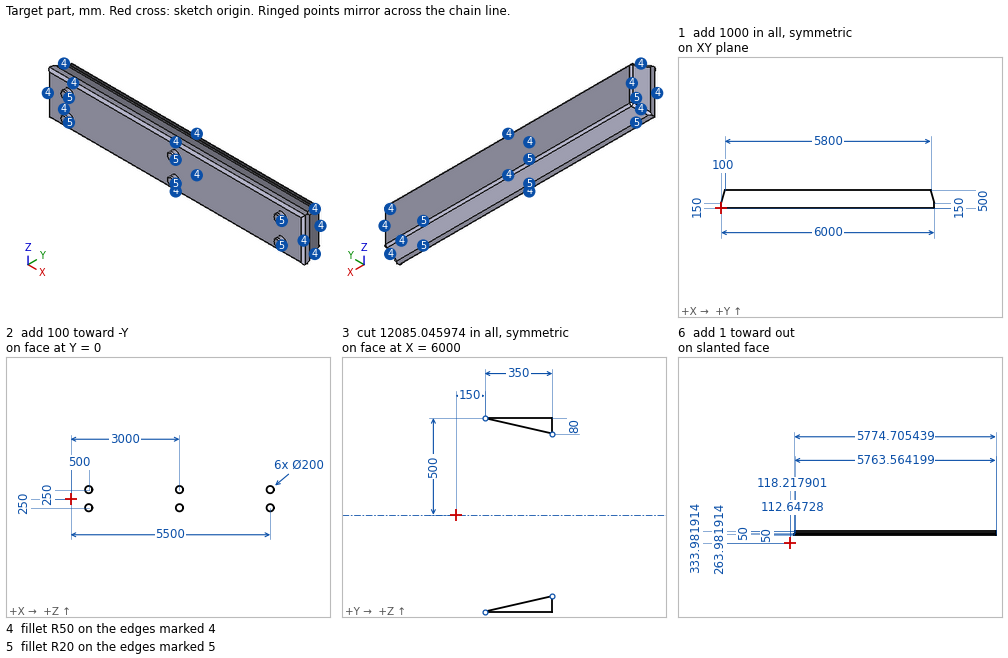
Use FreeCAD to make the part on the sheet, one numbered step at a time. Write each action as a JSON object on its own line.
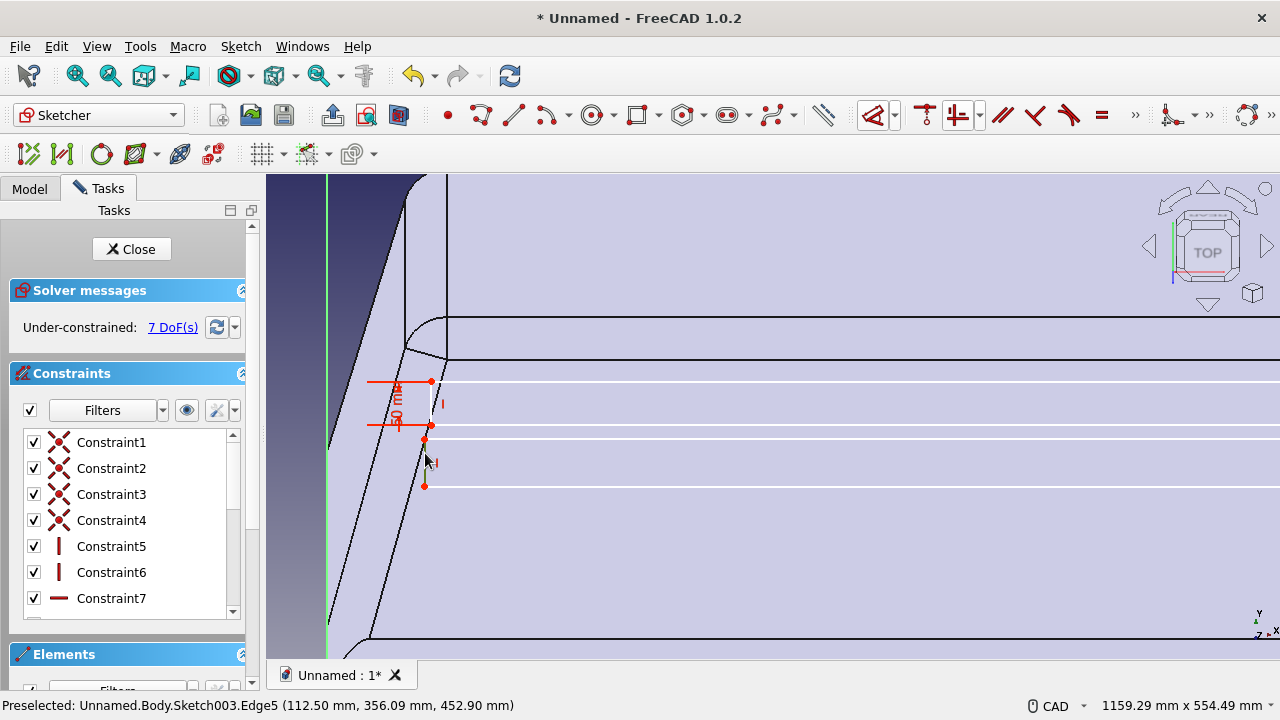
{"action": "left_click", "coordinate": [894, 116]}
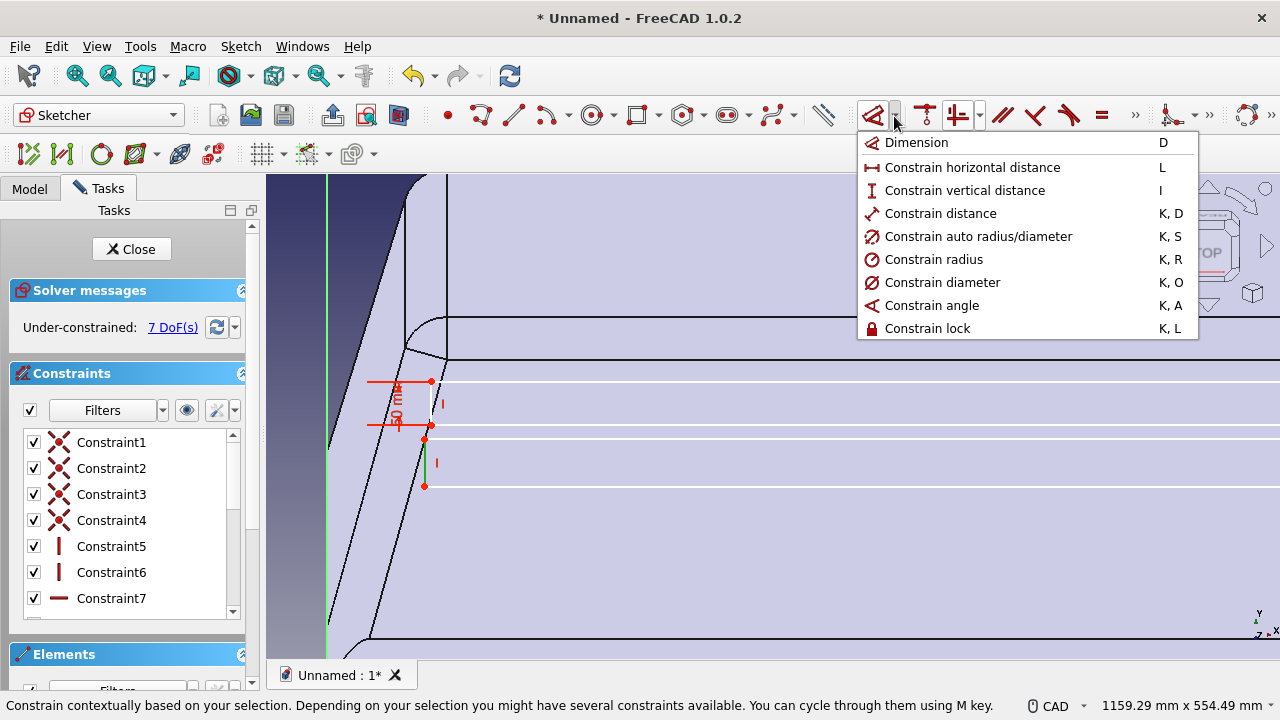
{"action": "left_click", "coordinate": [1028, 190]}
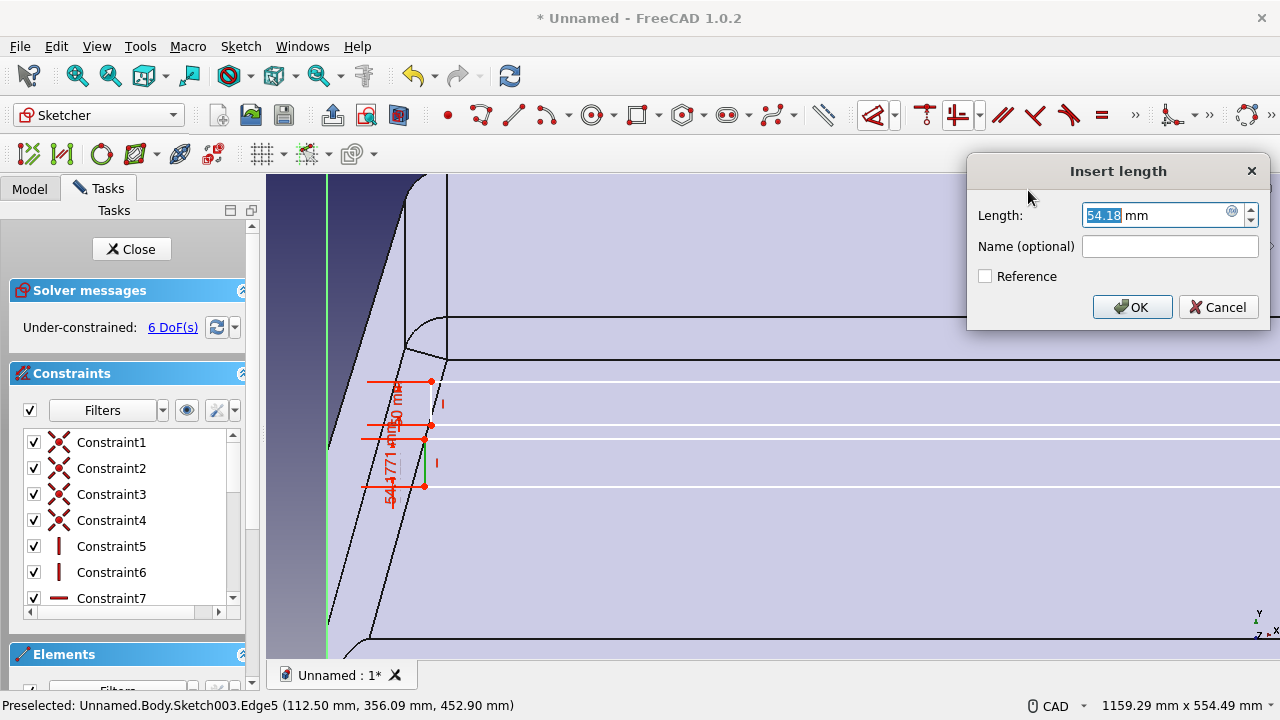
{"action": "type", "text": "50"}
{"action": "key", "text": "Return"}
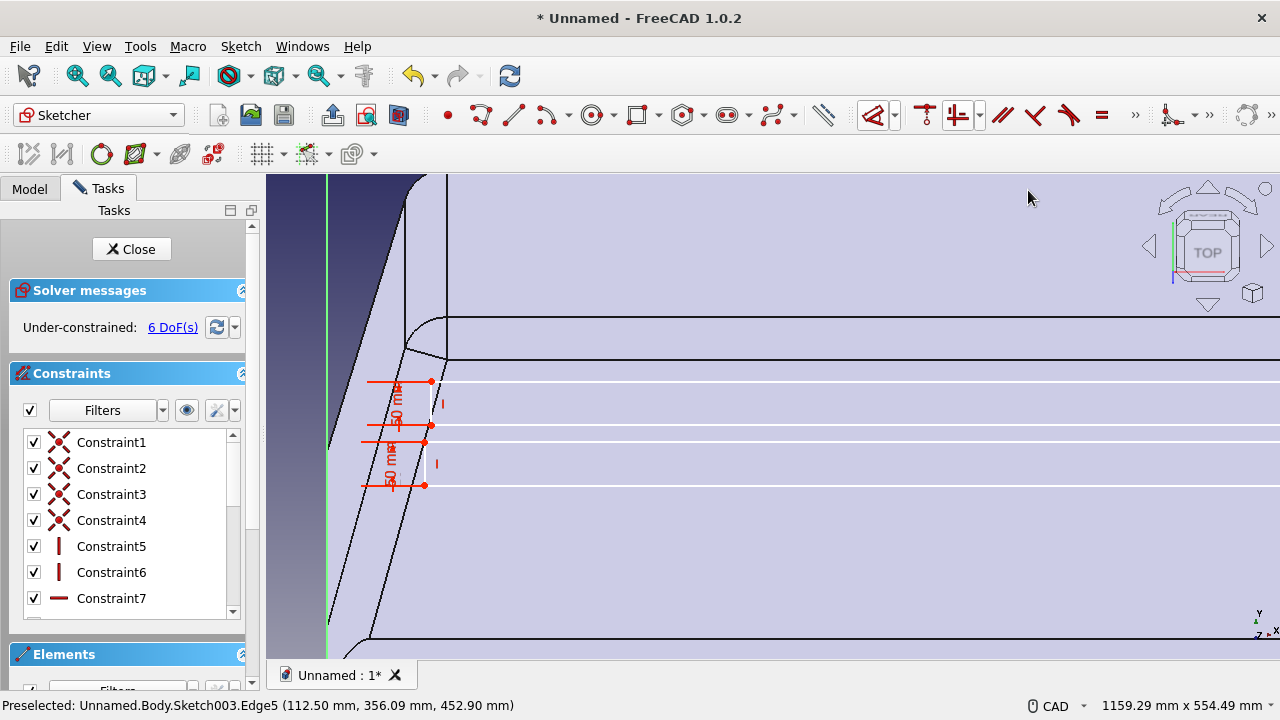
{"action": "left_click", "coordinate": [425, 442]}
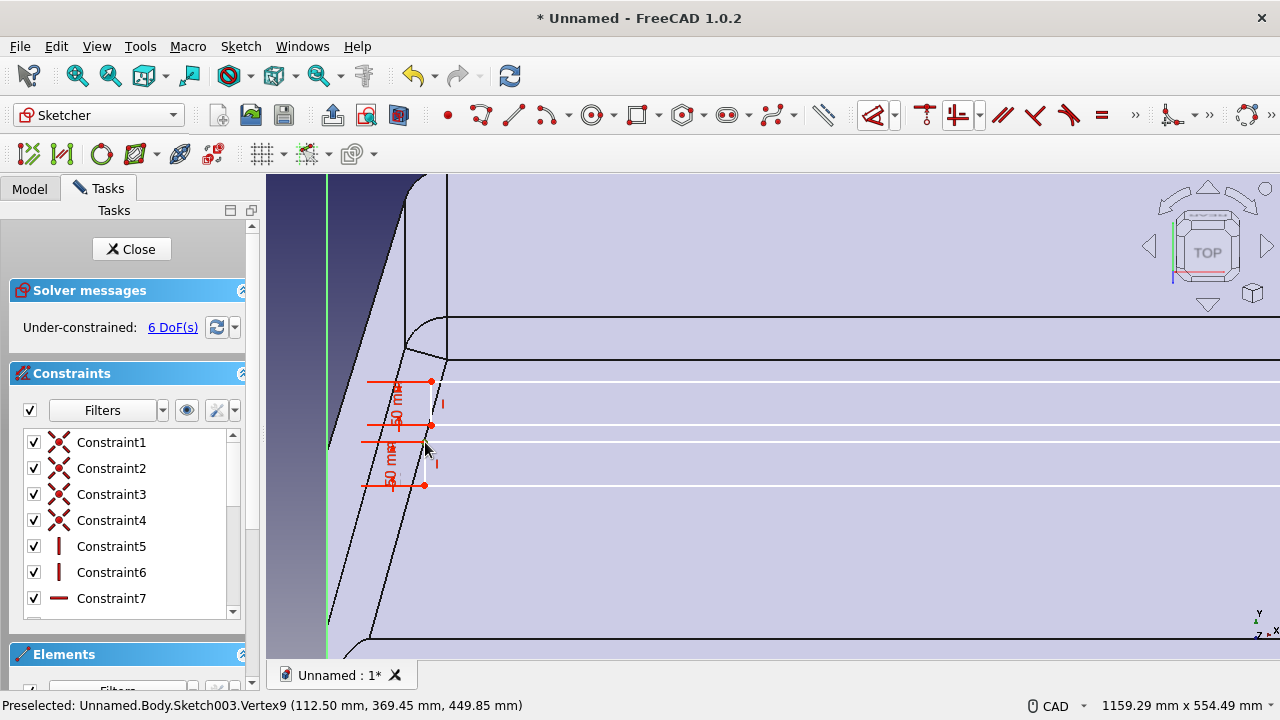
{"action": "key", "text": "l"}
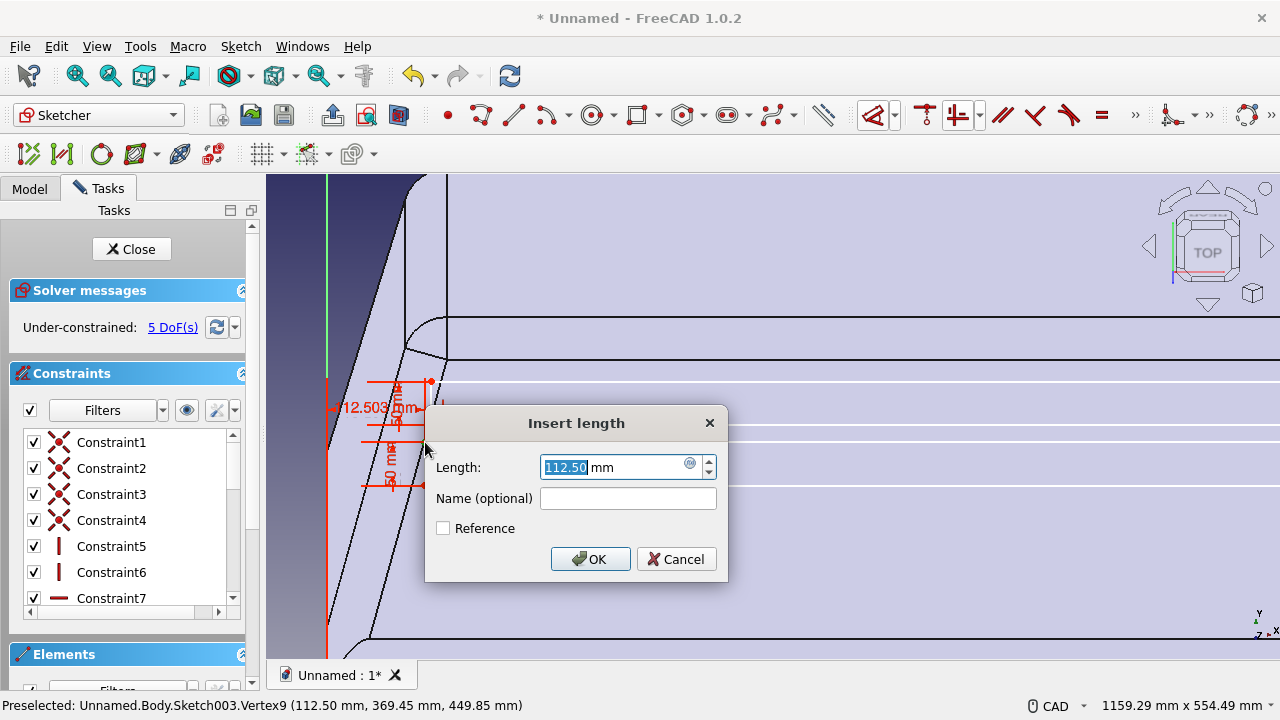
{"action": "type", "text": "112.64728"}
{"action": "key", "text": "Return"}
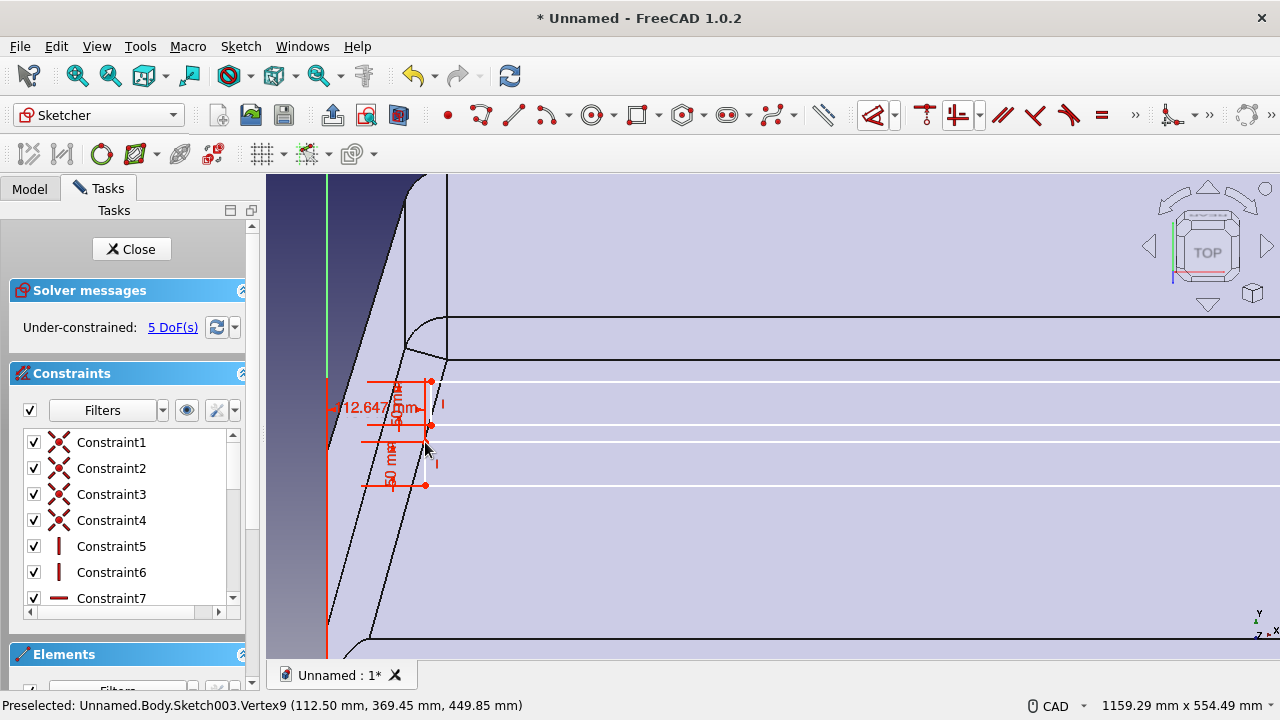
{"action": "scroll", "coordinate": [431, 403], "scroll_direction": "down", "scroll_amount": 11}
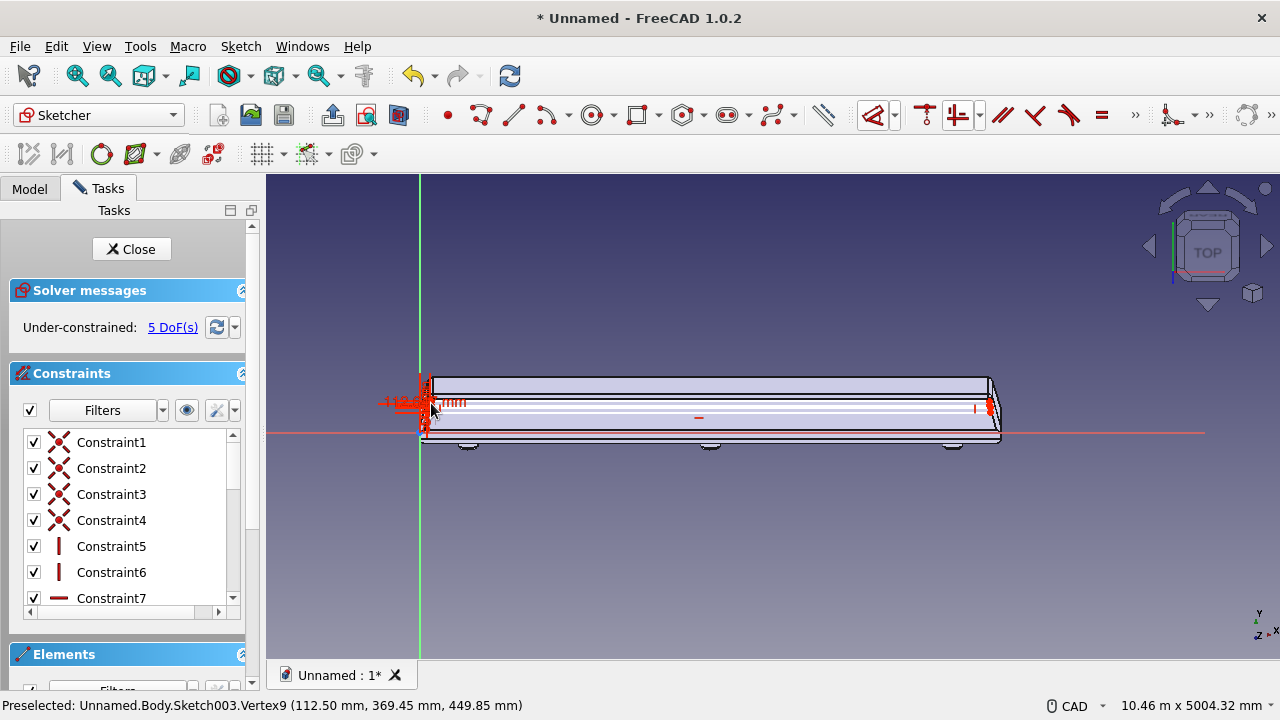
{"action": "scroll", "coordinate": [599, 406], "scroll_direction": "up", "scroll_amount": 11}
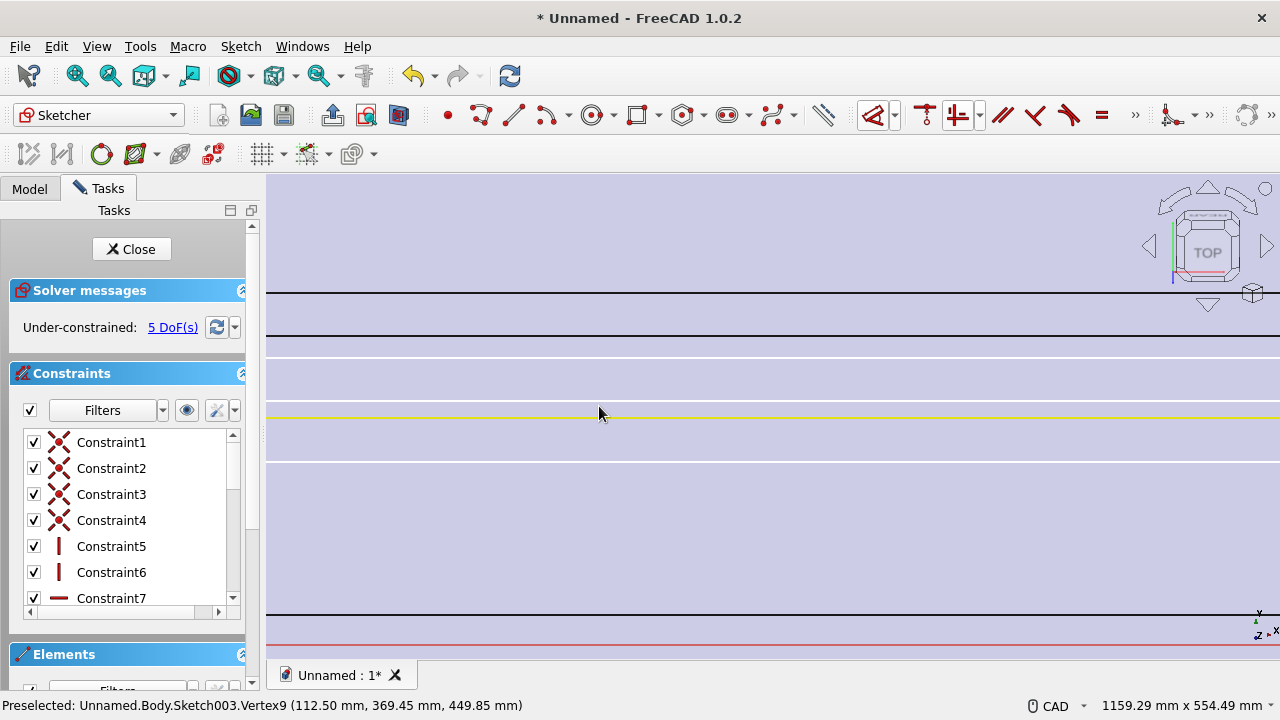
{"action": "left_click", "coordinate": [595, 401]}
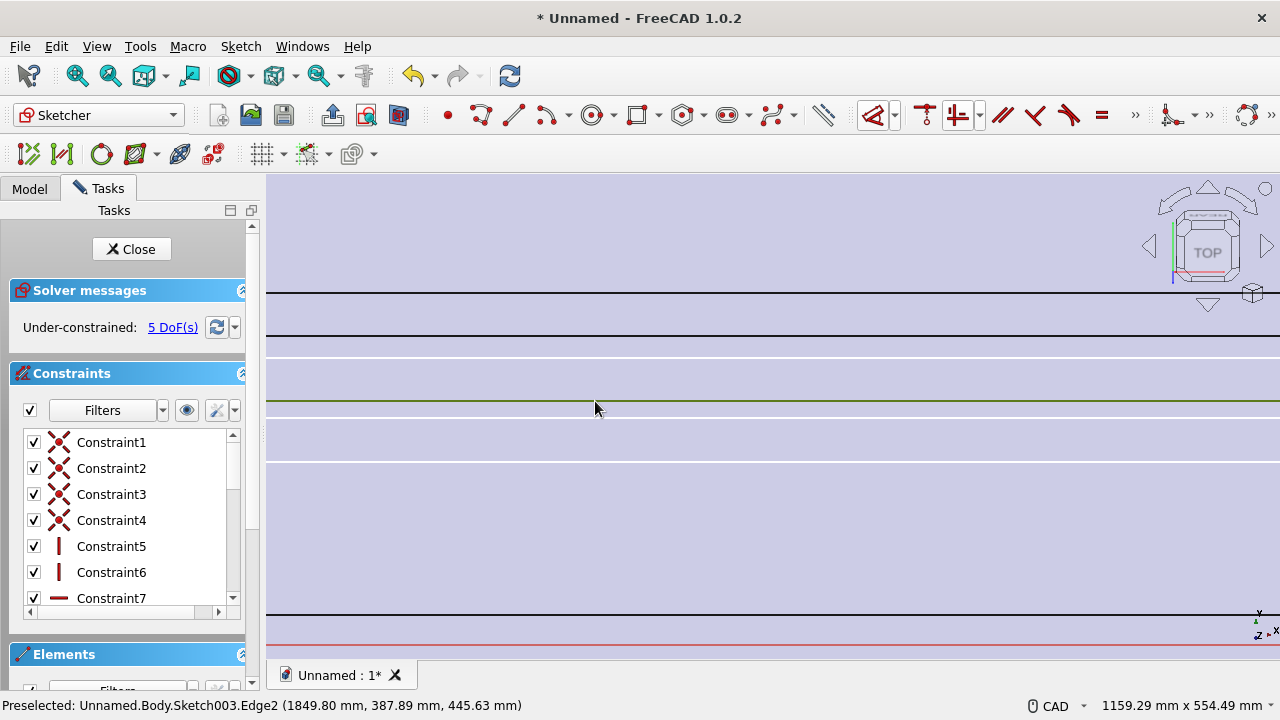
{"action": "key", "text": "l"}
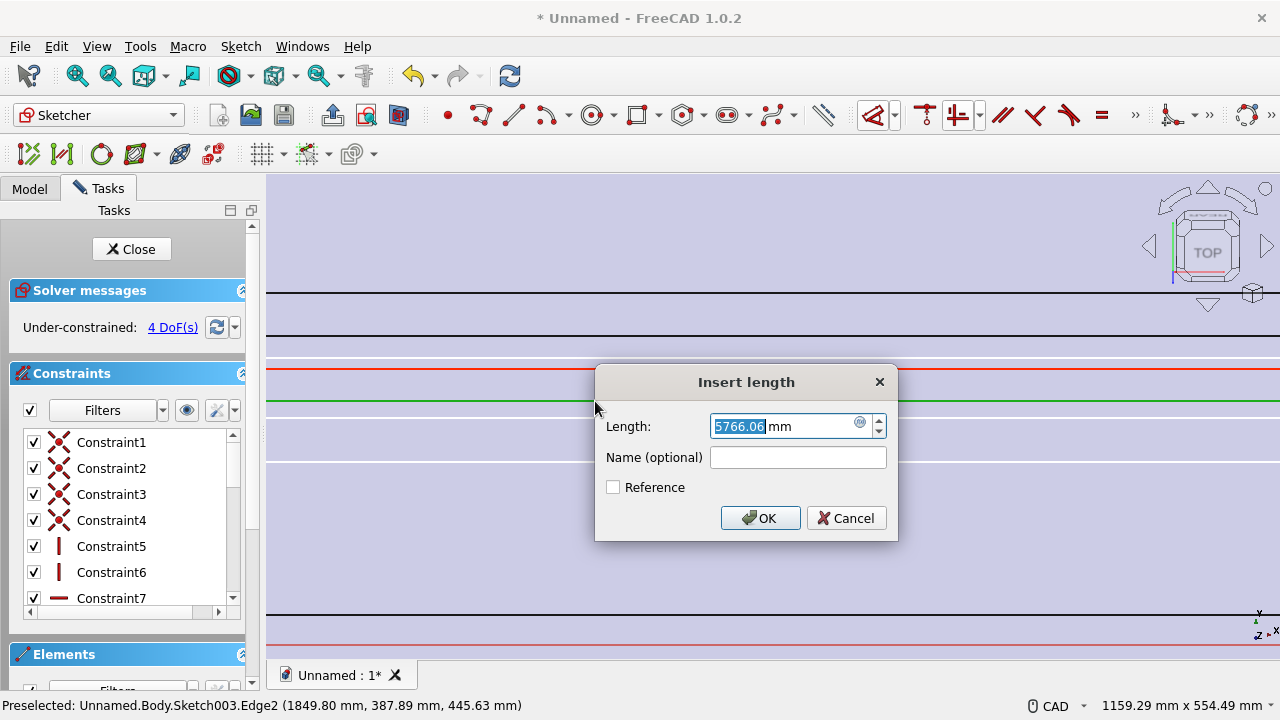
{"action": "type", "text": "5763.564199"}
{"action": "key", "text": "Return"}